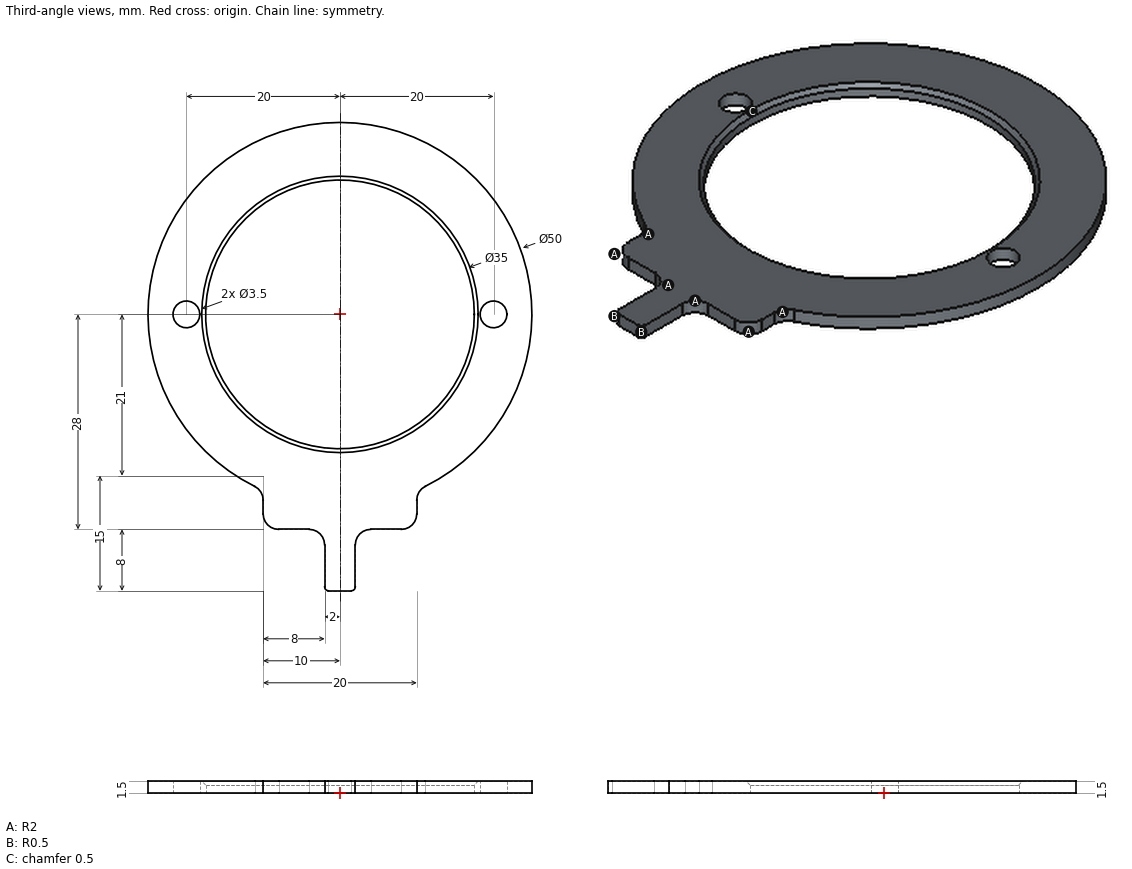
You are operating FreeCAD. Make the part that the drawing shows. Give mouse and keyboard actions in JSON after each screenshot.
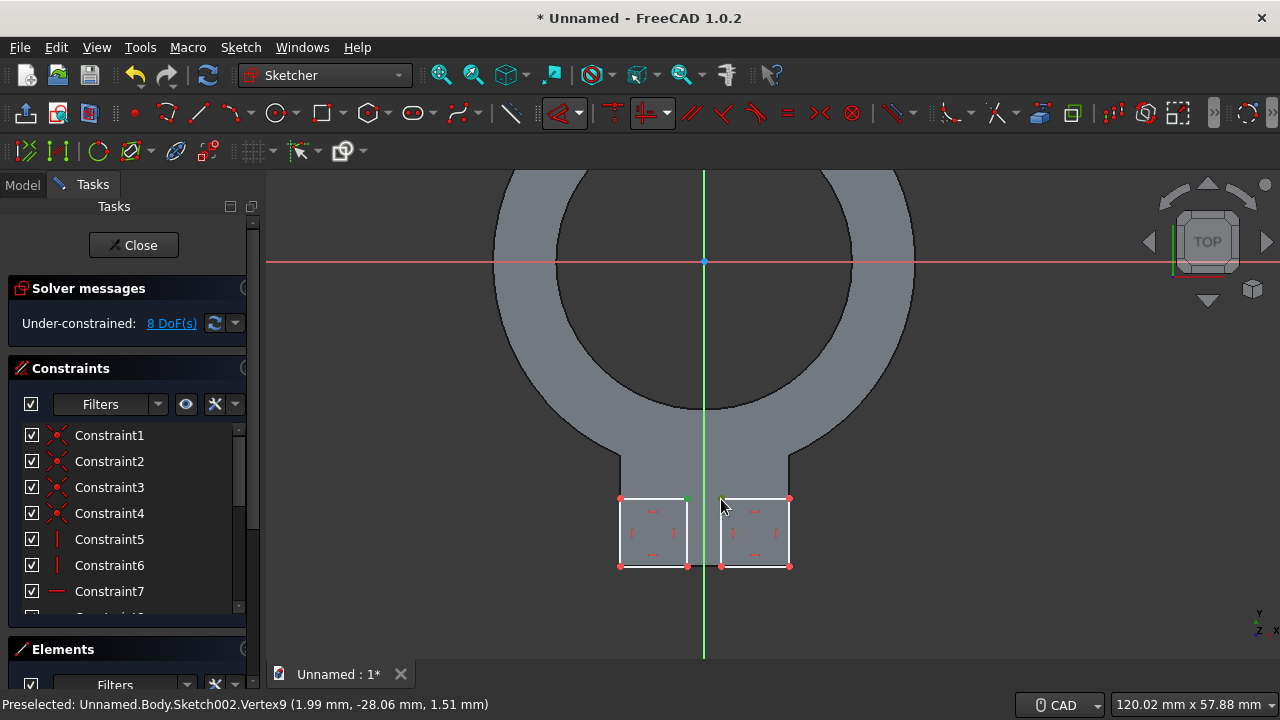
{"action": "left_click", "coordinate": [704, 600]}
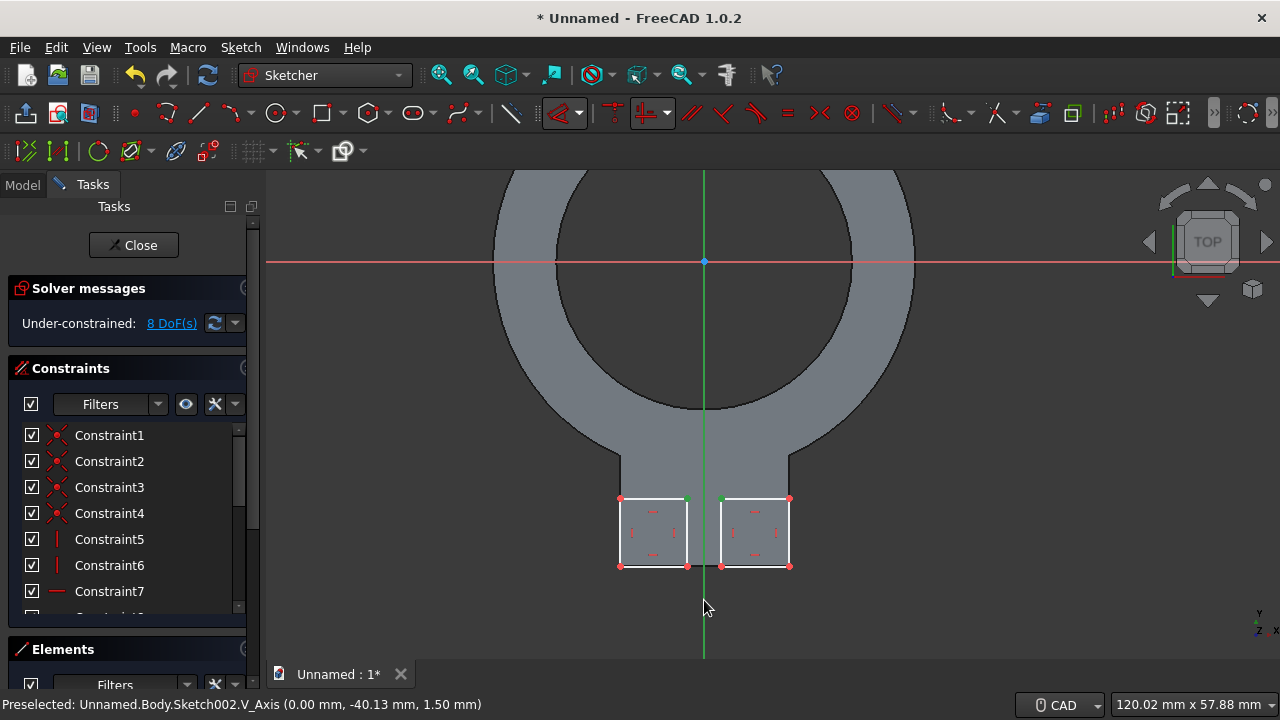
{"action": "left_click", "coordinate": [820, 114]}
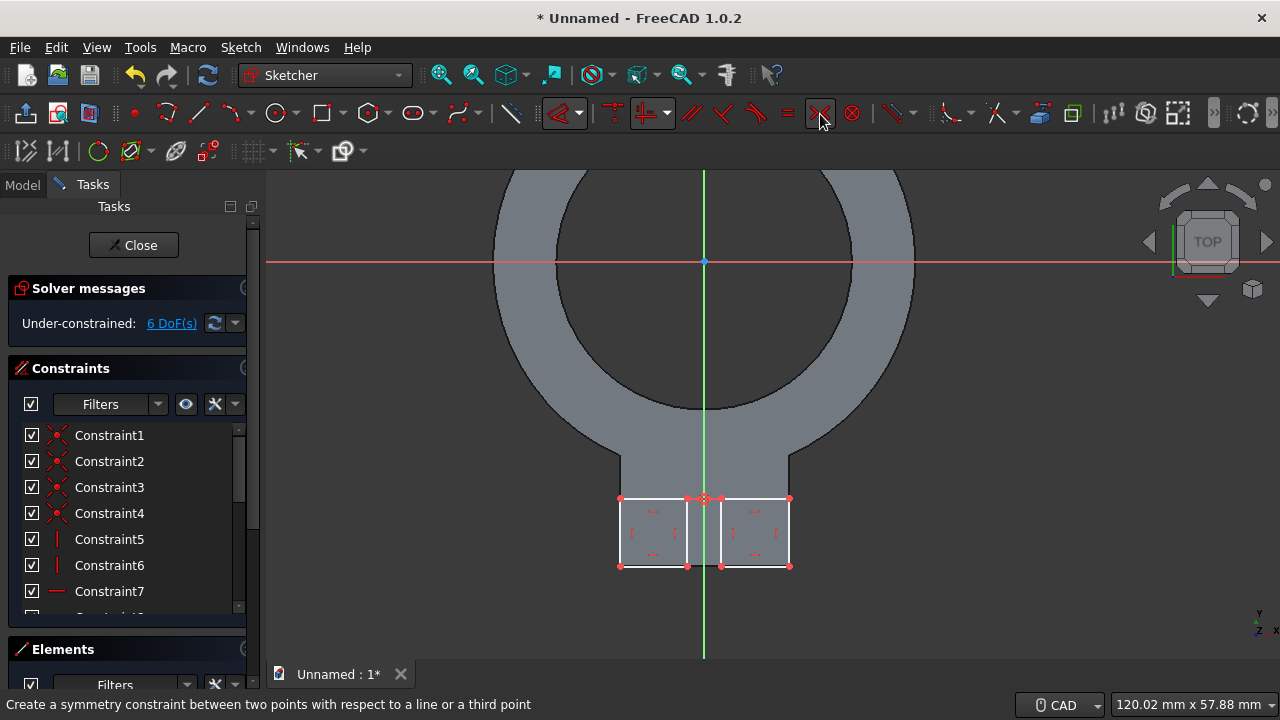
{"action": "left_click", "coordinate": [620, 567]}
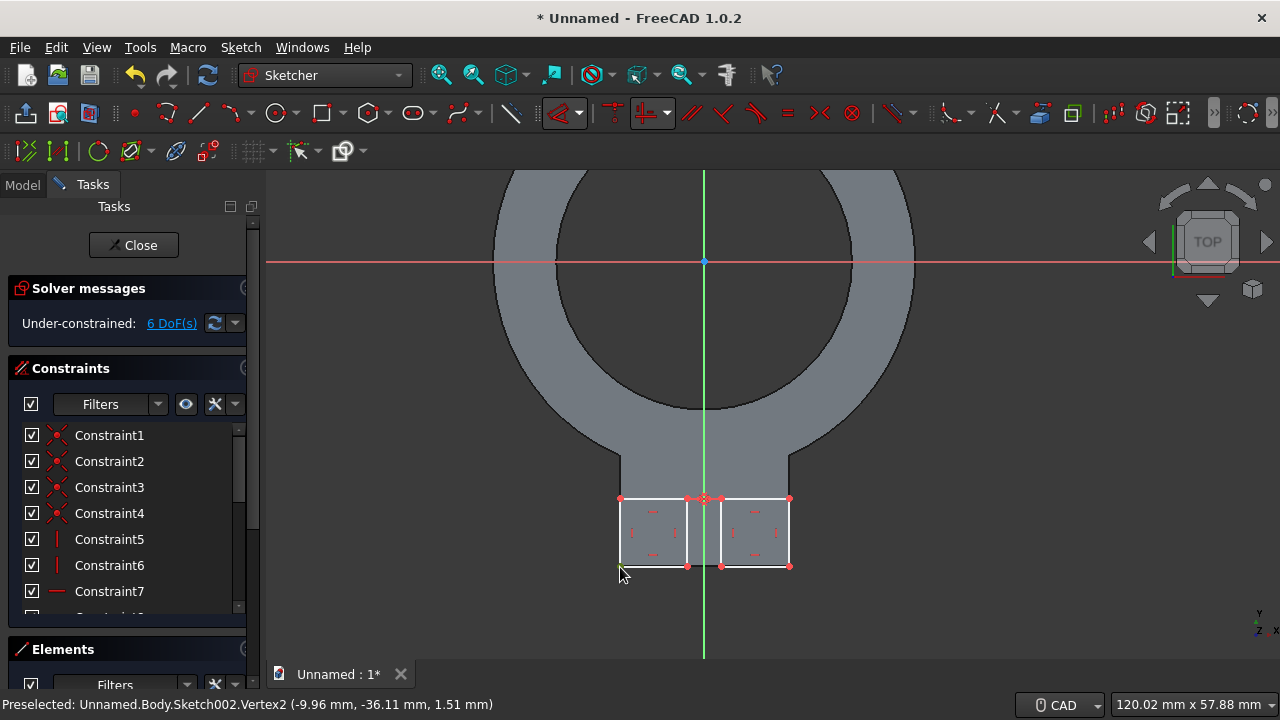
{"action": "left_click", "coordinate": [789, 567]}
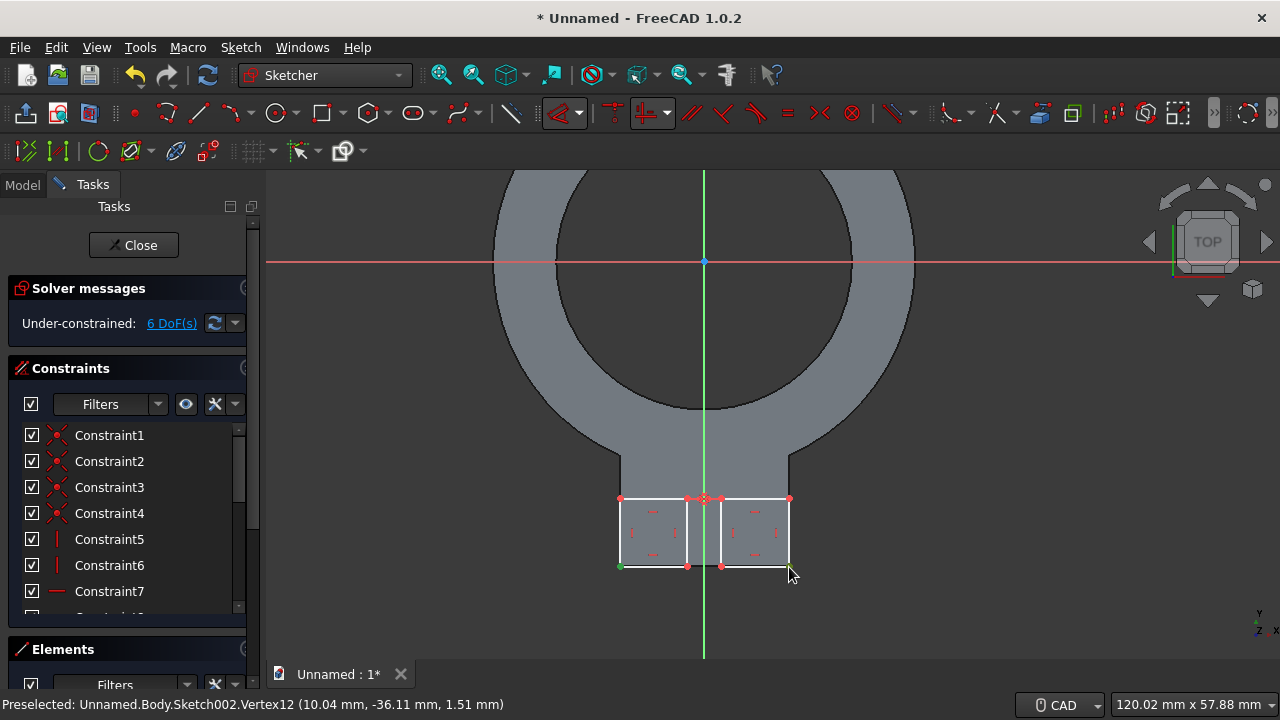
{"action": "left_click", "coordinate": [704, 600]}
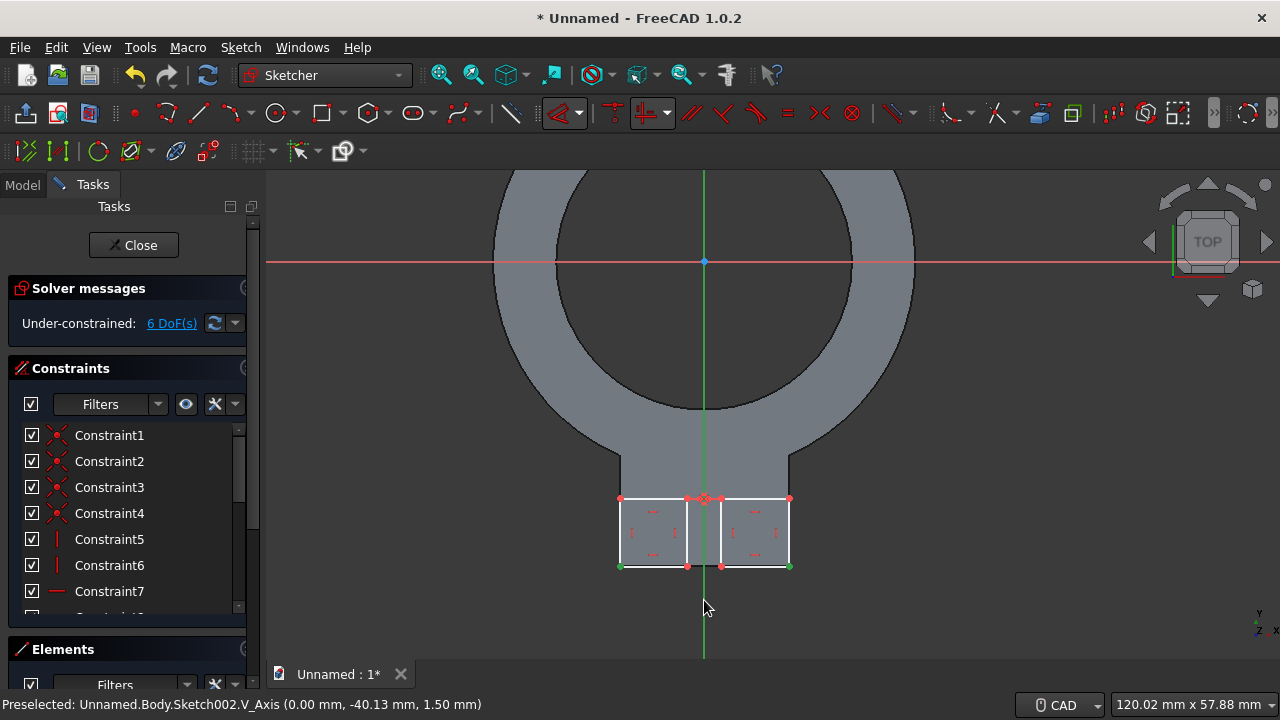
{"action": "left_click", "coordinate": [820, 114]}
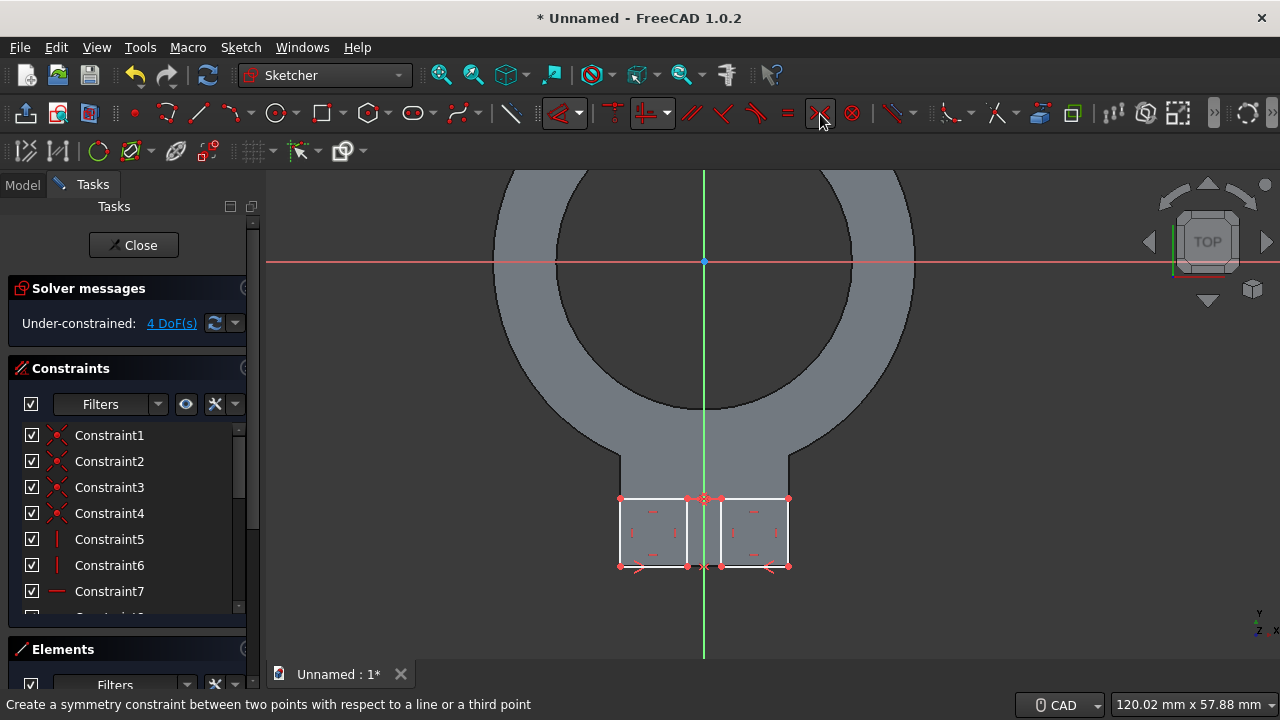
{"action": "left_click", "coordinate": [620, 519]}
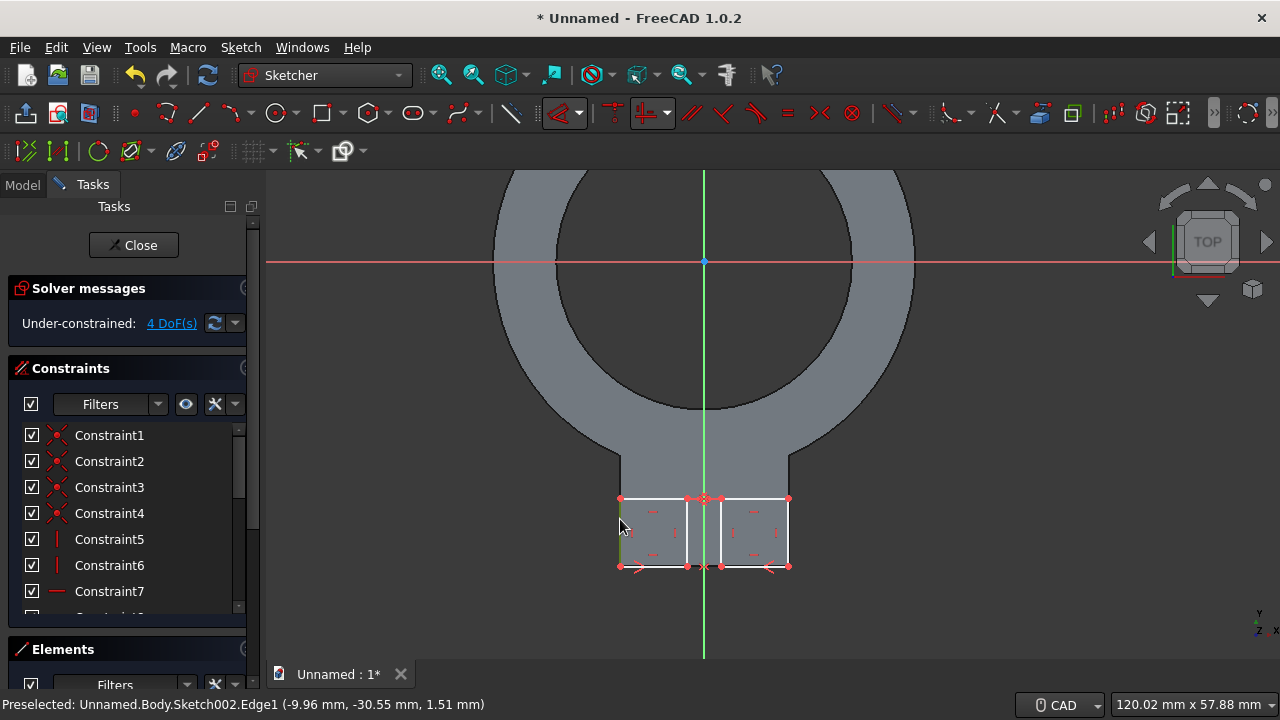
{"action": "key", "text": "i"}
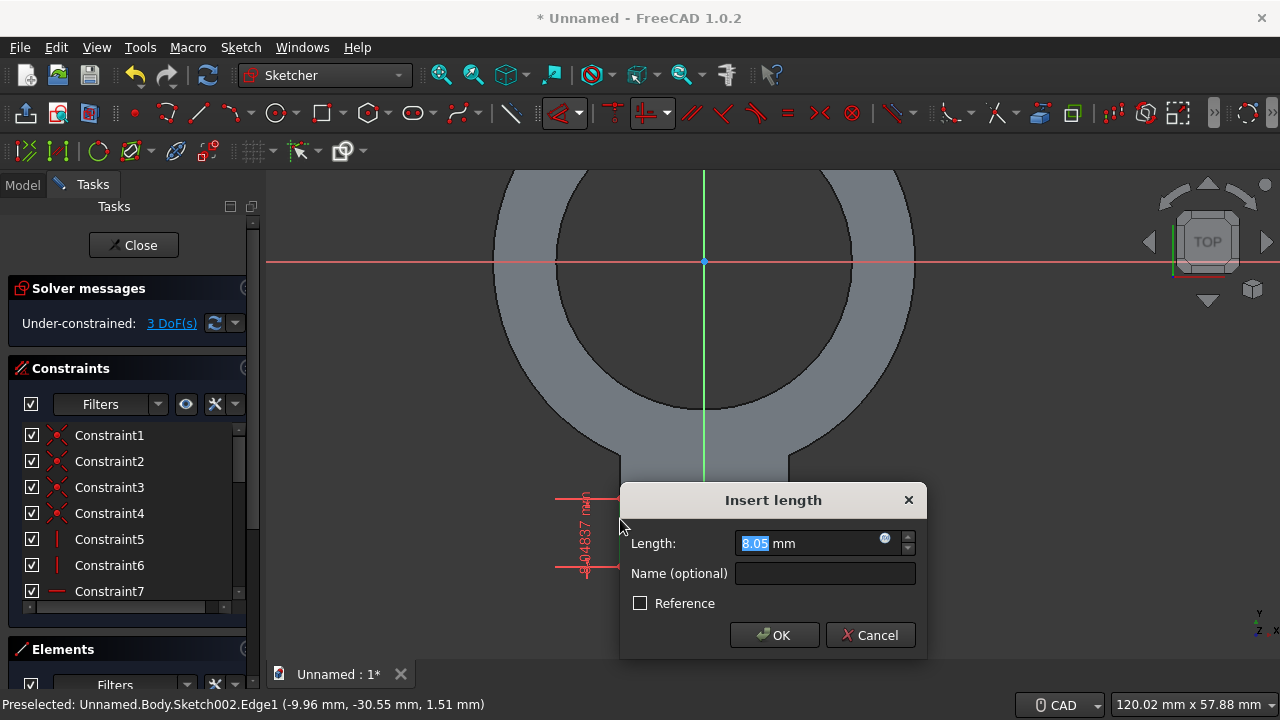
{"action": "type", "text": "8"}
{"action": "key", "text": "Return"}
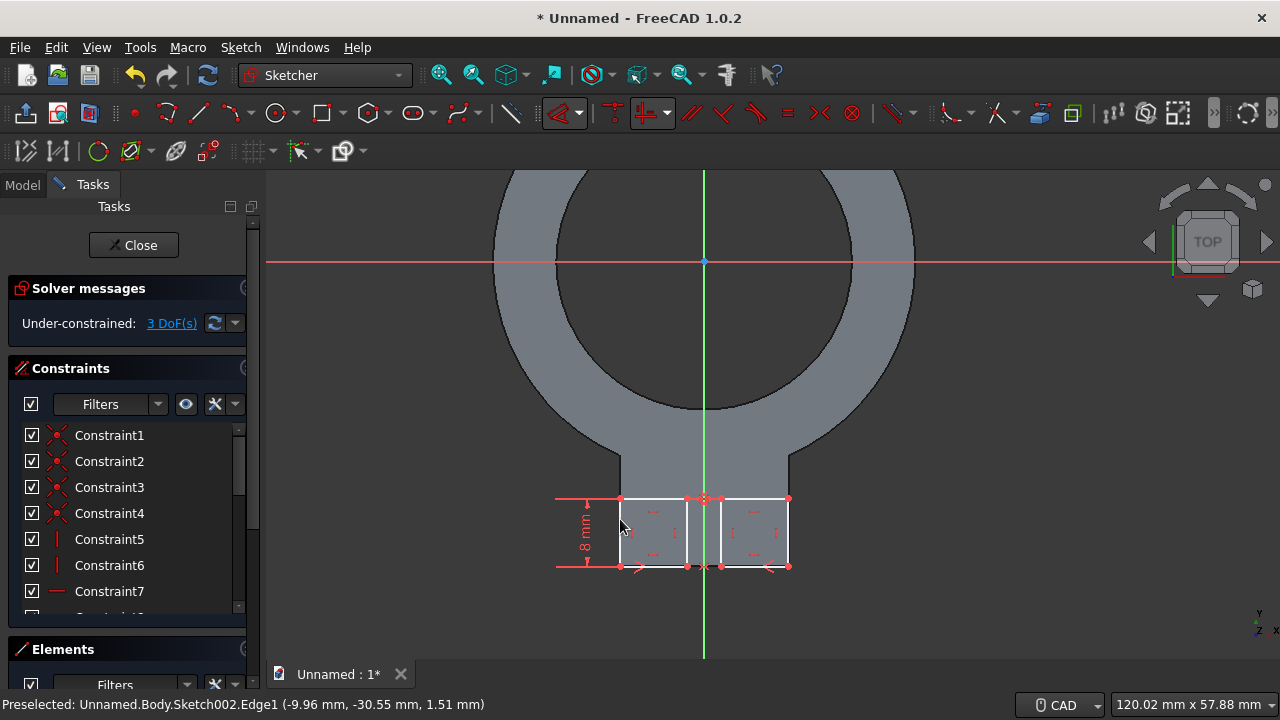
{"action": "left_click", "coordinate": [640, 567]}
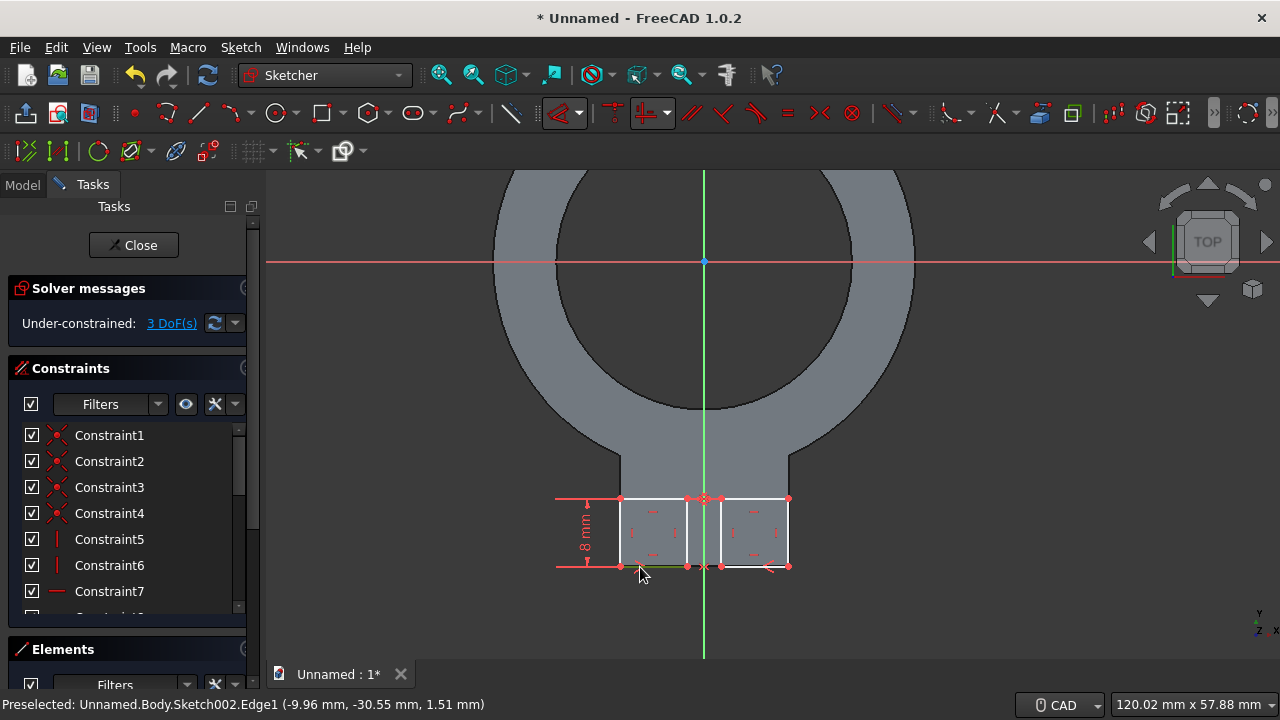
{"action": "left_click", "coordinate": [582, 114]}